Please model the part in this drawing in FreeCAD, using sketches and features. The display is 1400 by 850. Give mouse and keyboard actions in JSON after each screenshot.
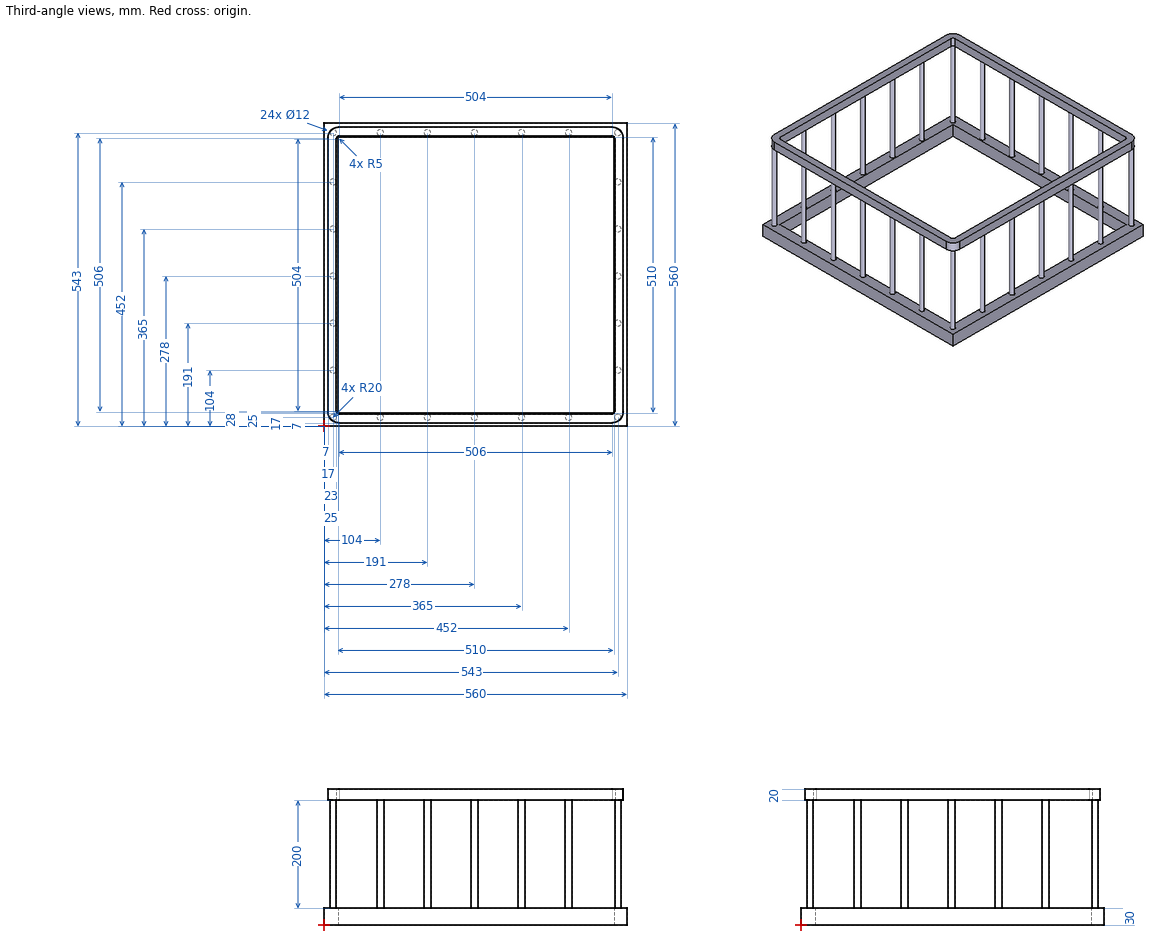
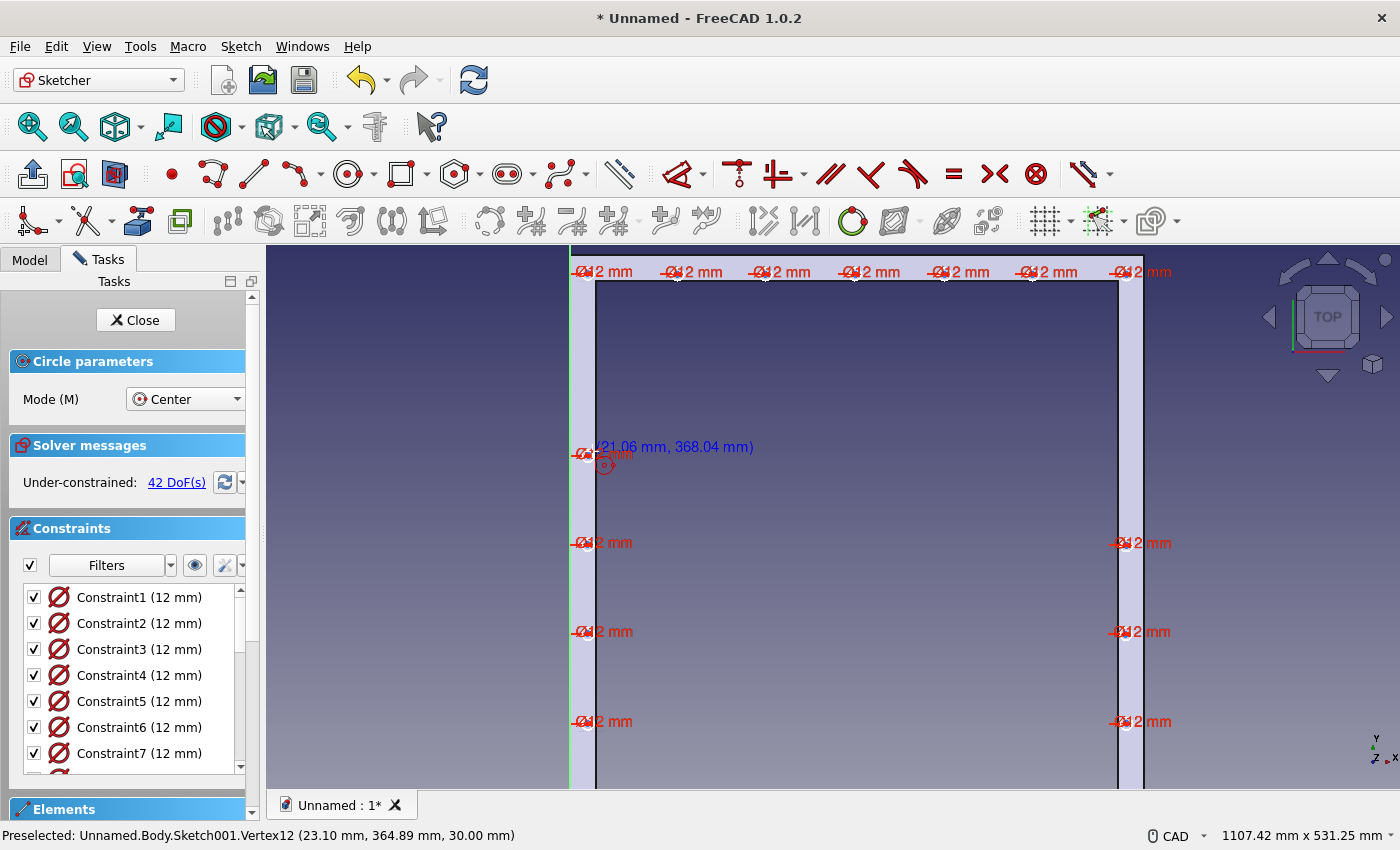
{"action": "scroll", "coordinate": [1126, 455], "scroll_direction": "up", "scroll_amount": 7}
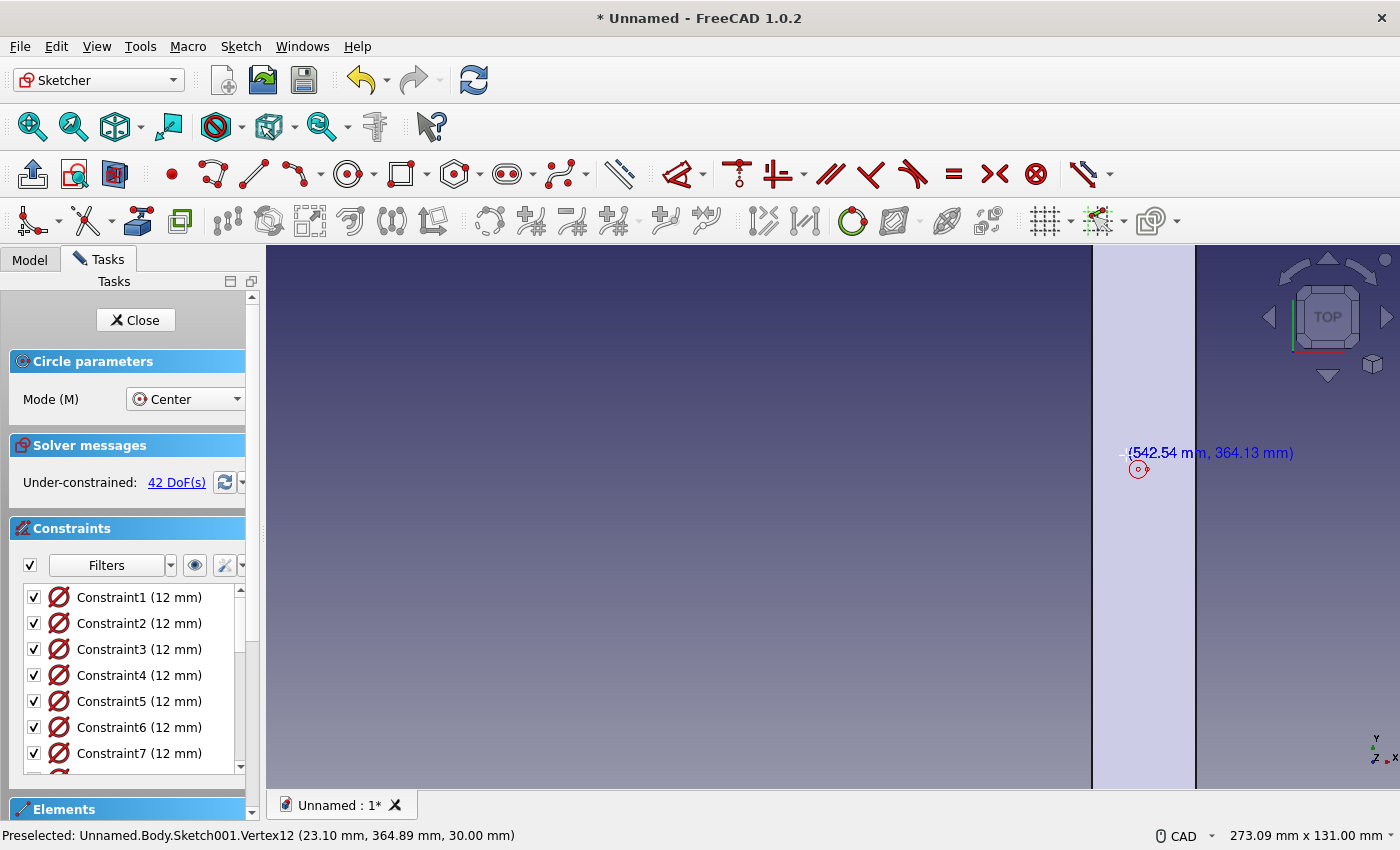
{"action": "scroll", "coordinate": [914, 455], "scroll_direction": "down", "scroll_amount": 9}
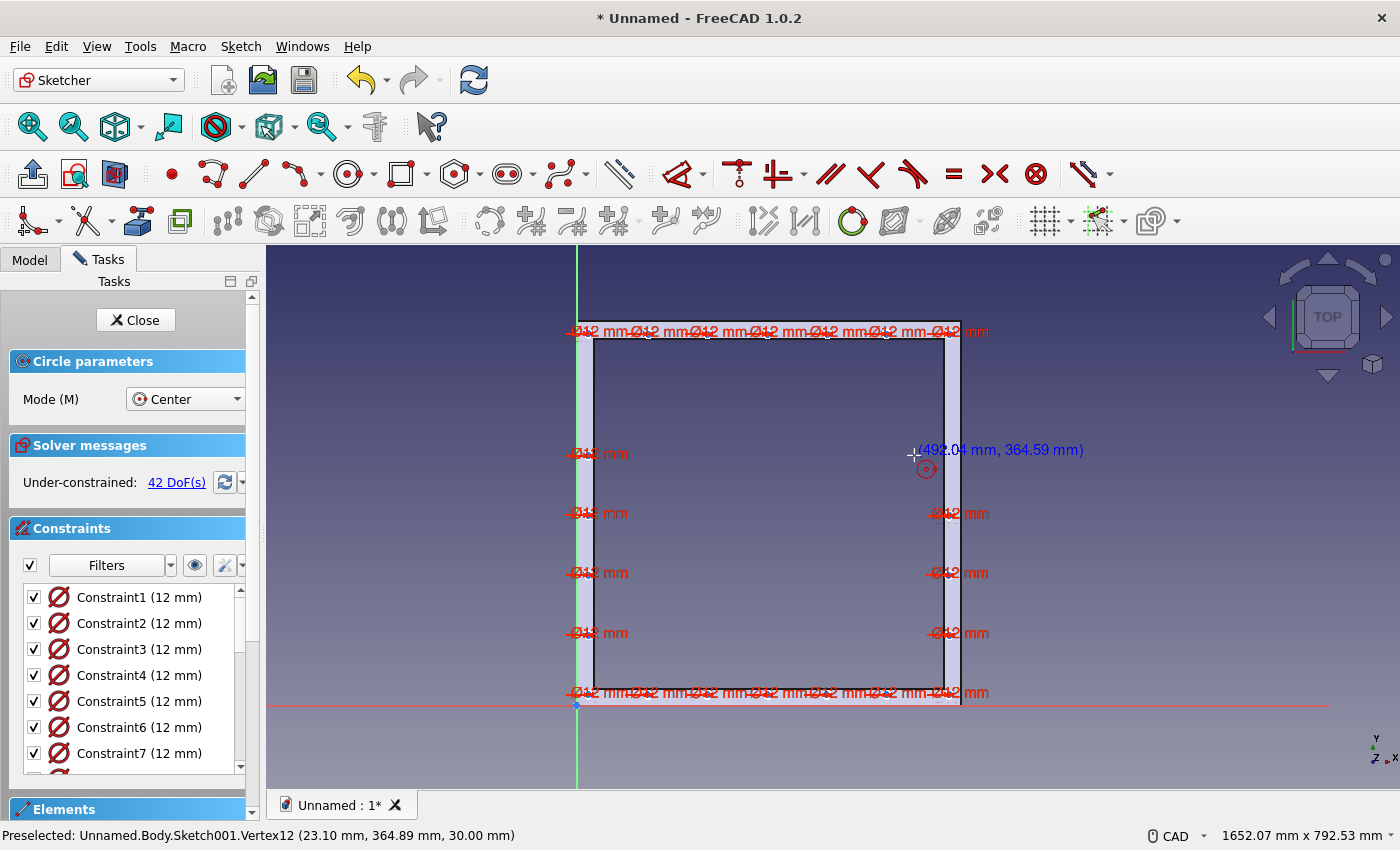
{"action": "left_click", "coordinate": [949, 455]}
{"action": "mouse_move", "coordinate": [952, 452]}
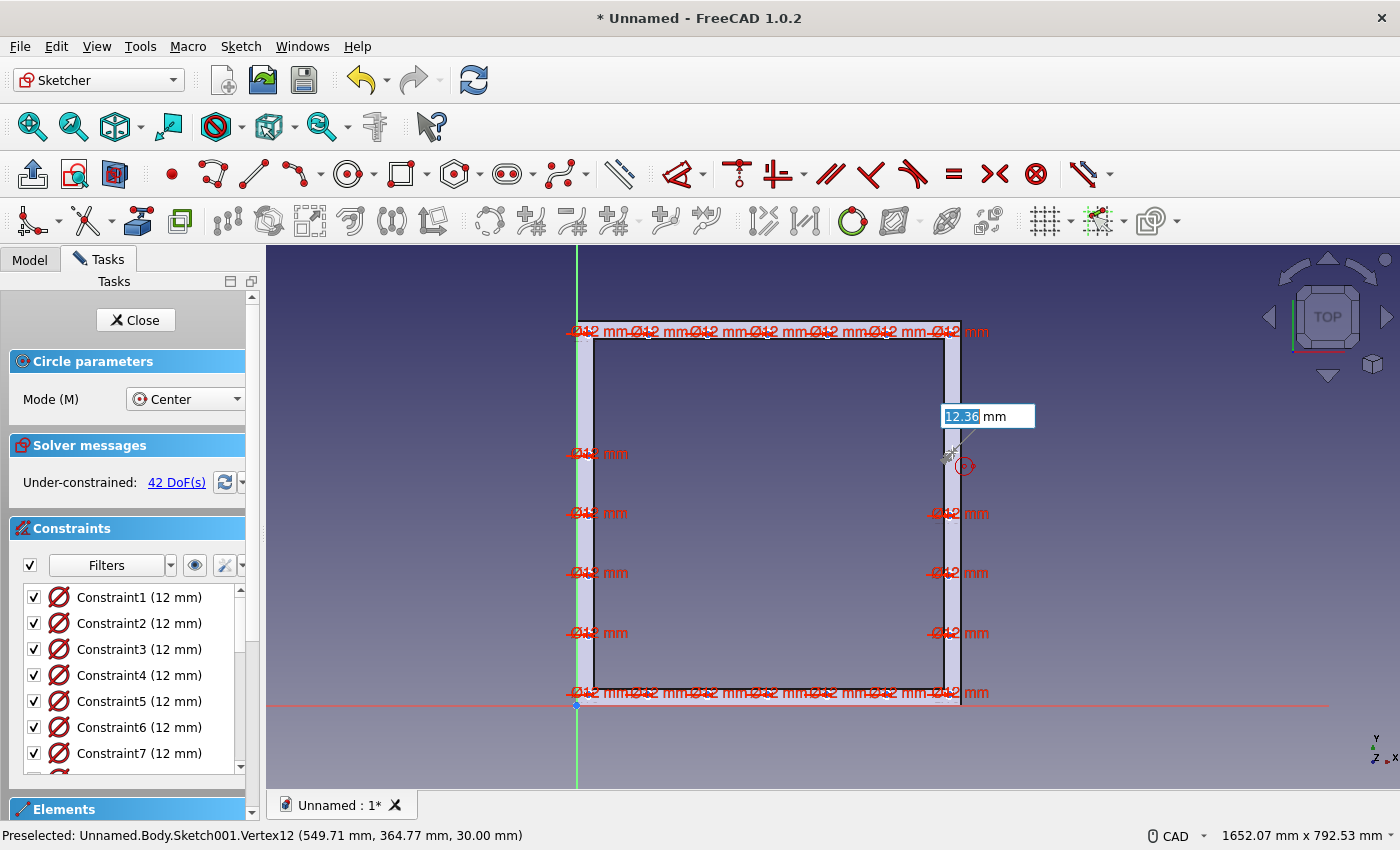
{"action": "type", "text": "12"}
{"action": "key", "text": "Return"}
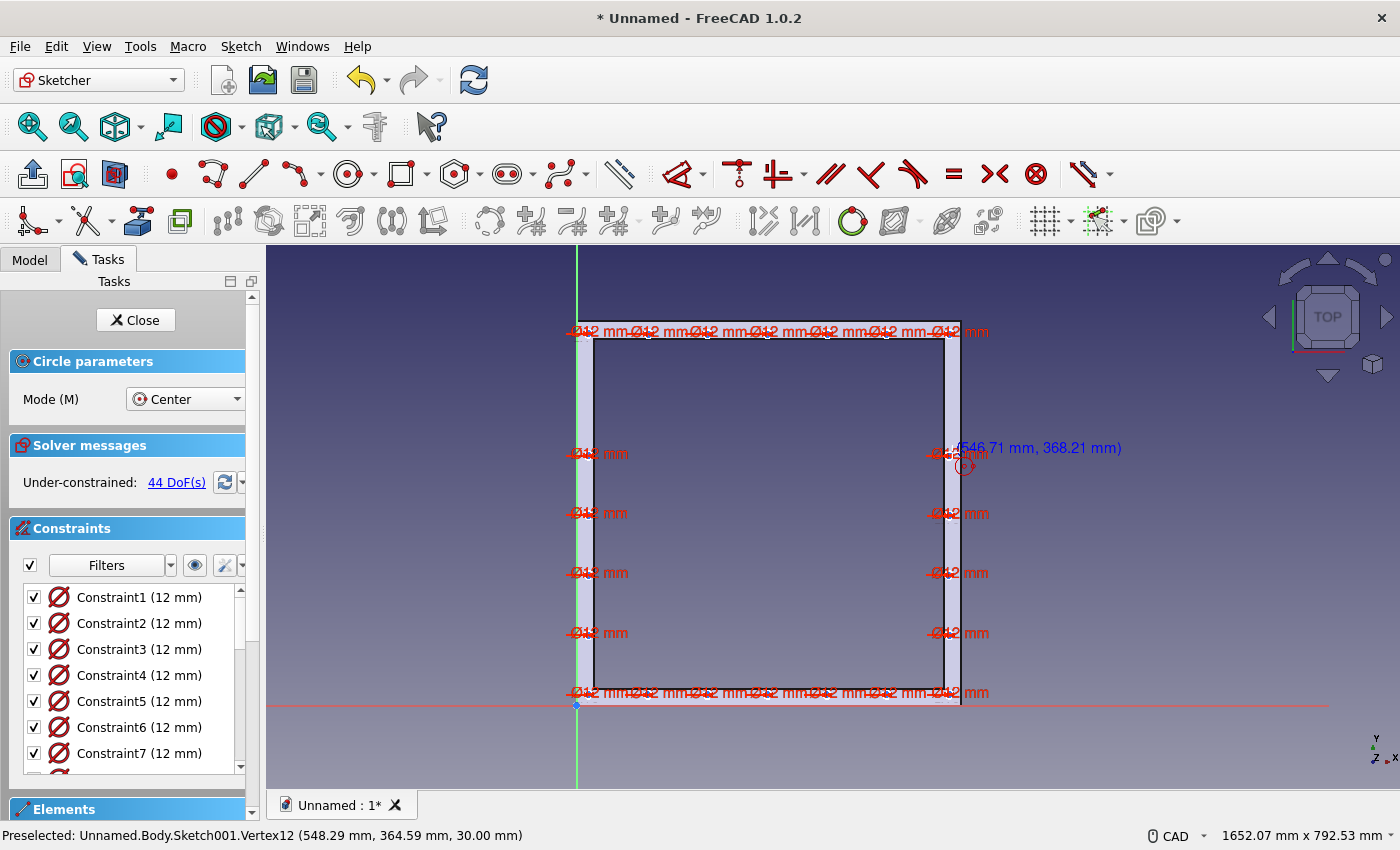
{"action": "scroll", "coordinate": [588, 395], "scroll_direction": "up", "scroll_amount": 9}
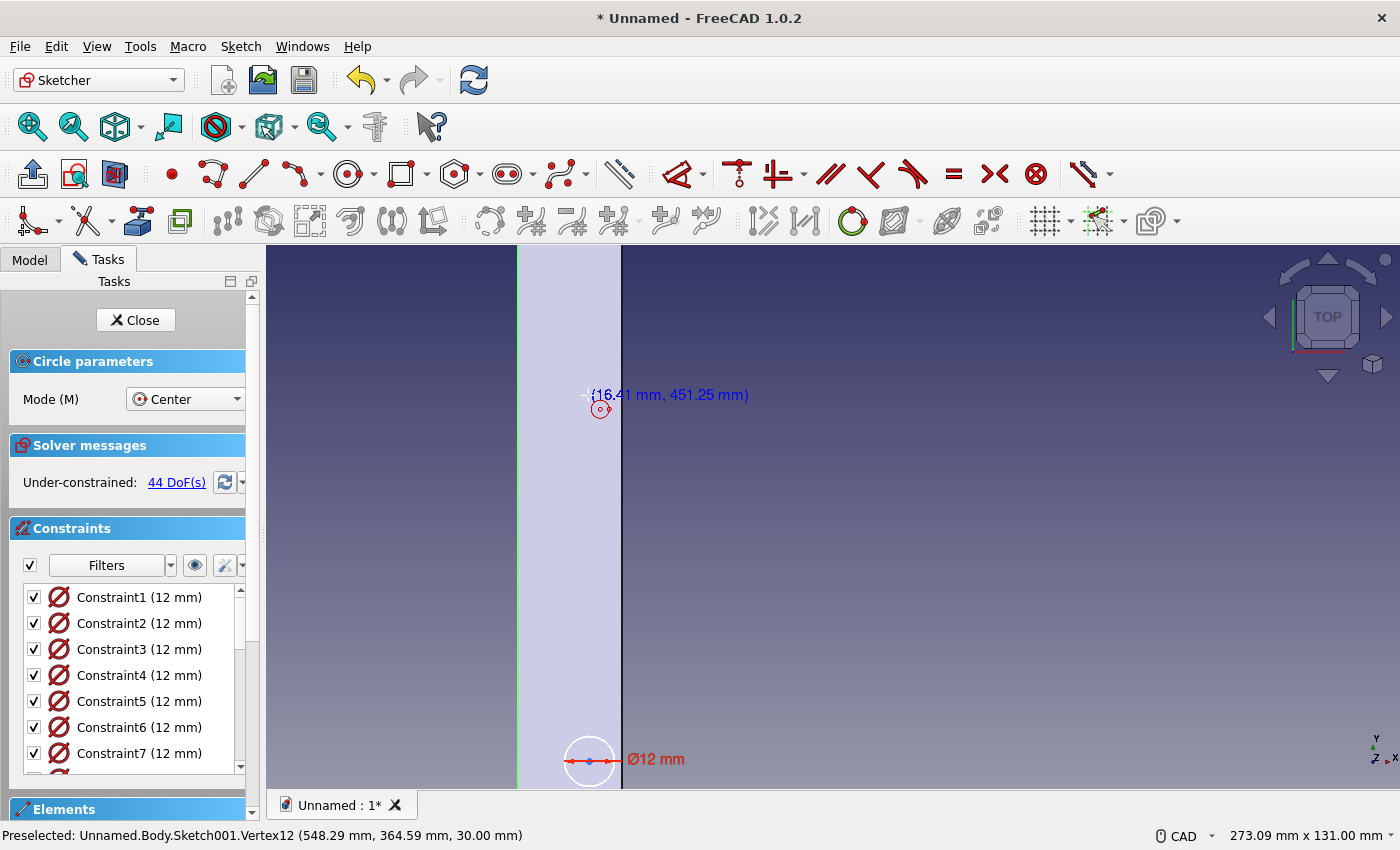
{"action": "scroll", "coordinate": [588, 395], "scroll_direction": "down", "scroll_amount": 9}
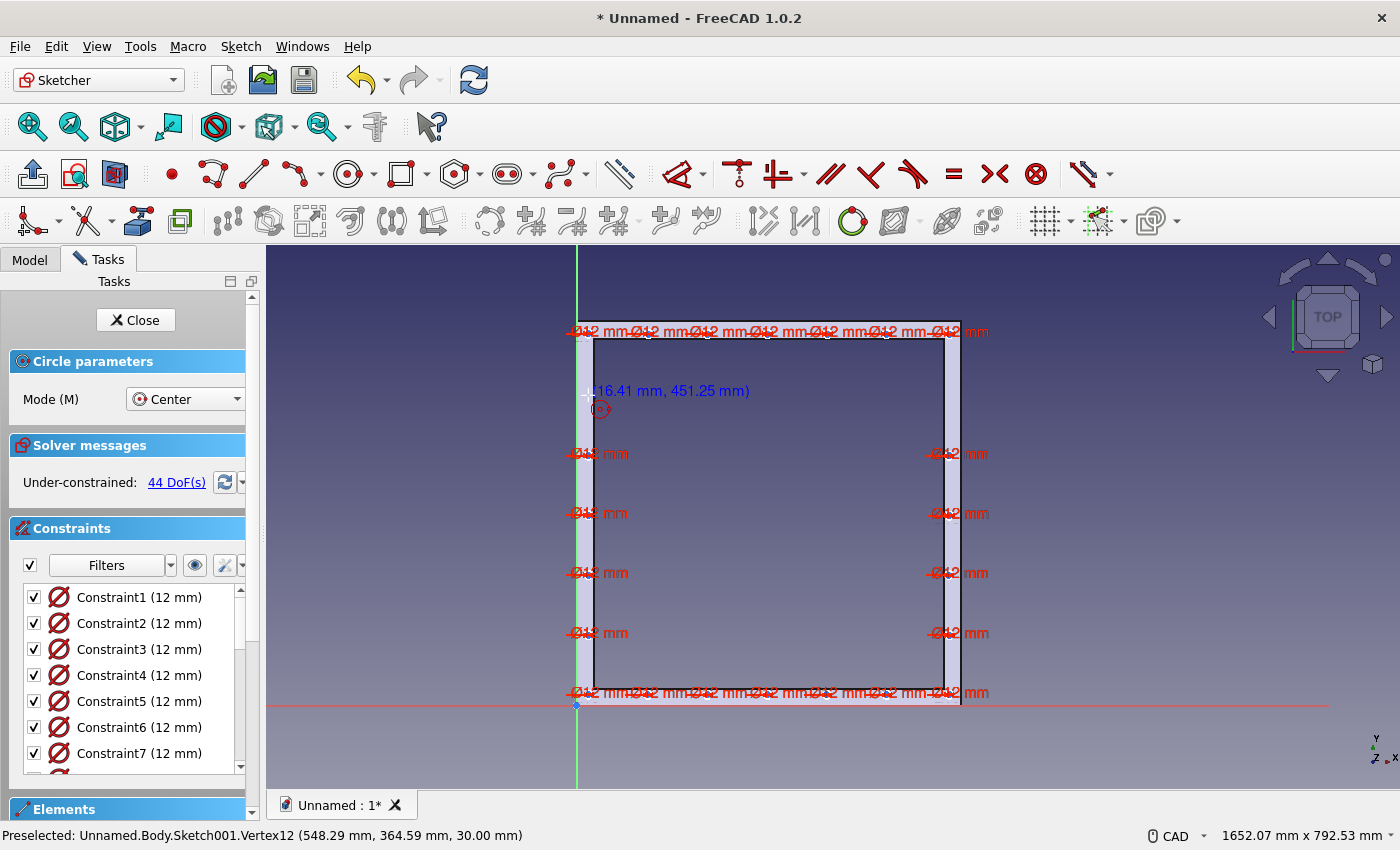
{"action": "scroll", "coordinate": [588, 395], "scroll_direction": "up", "scroll_amount": 2}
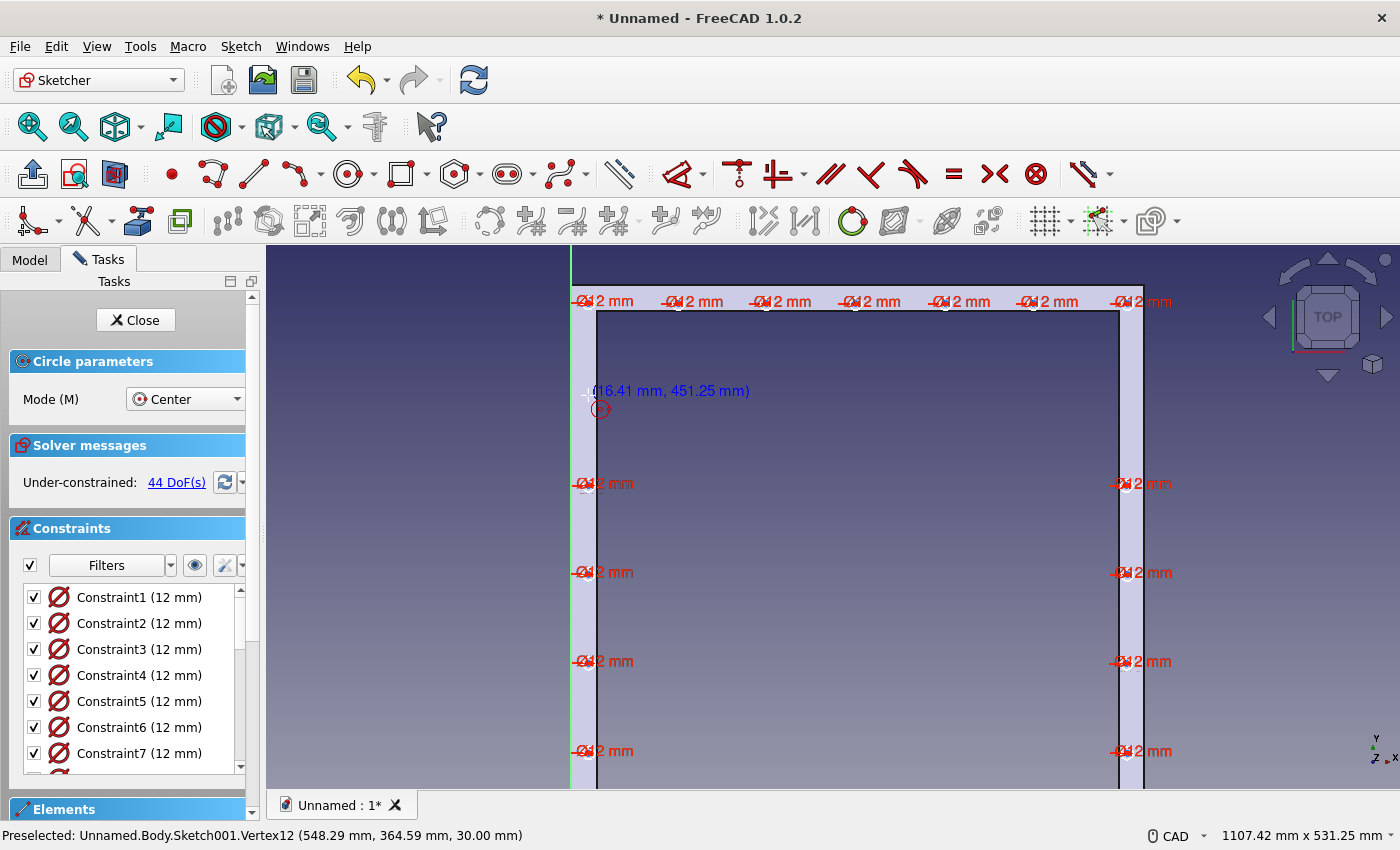
{"action": "left_click", "coordinate": [588, 396]}
{"action": "mouse_move", "coordinate": [593, 391]}